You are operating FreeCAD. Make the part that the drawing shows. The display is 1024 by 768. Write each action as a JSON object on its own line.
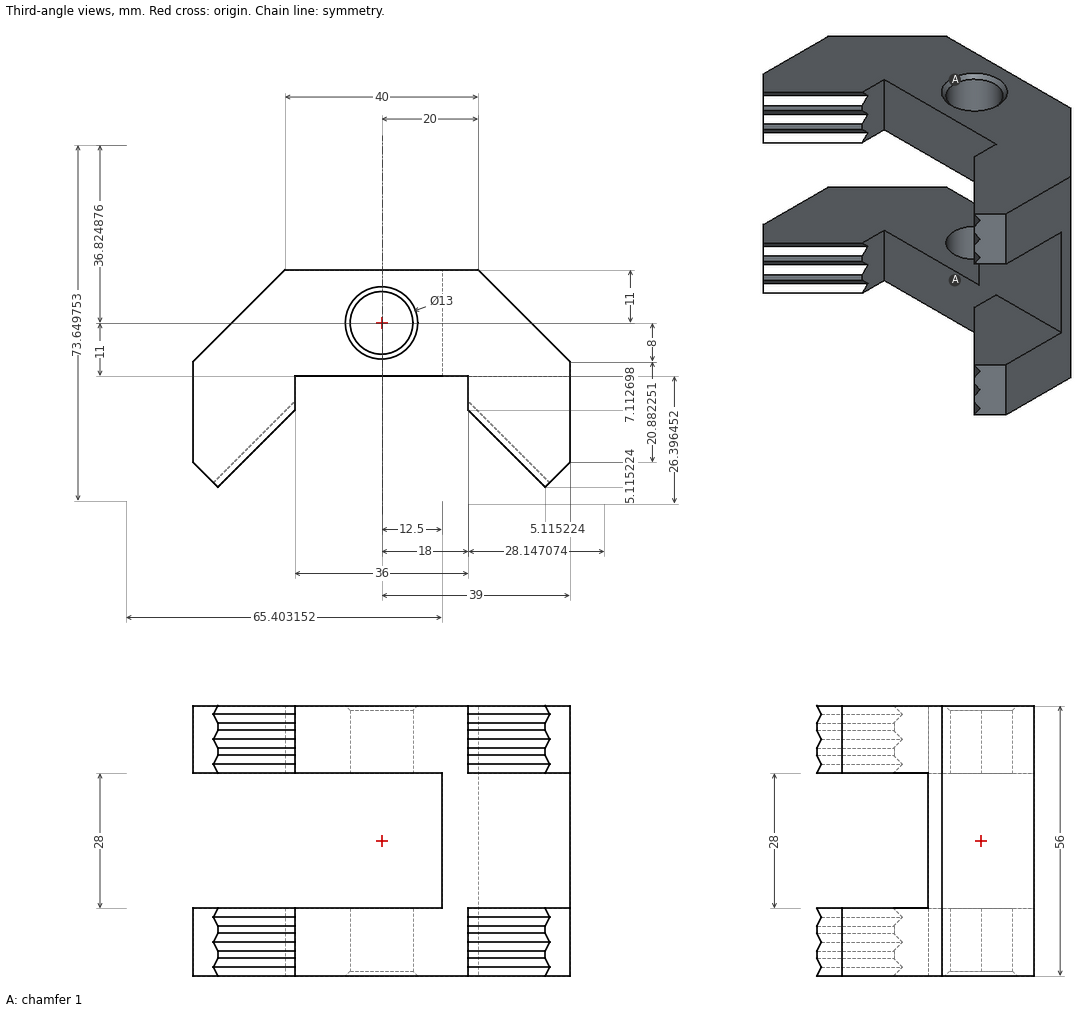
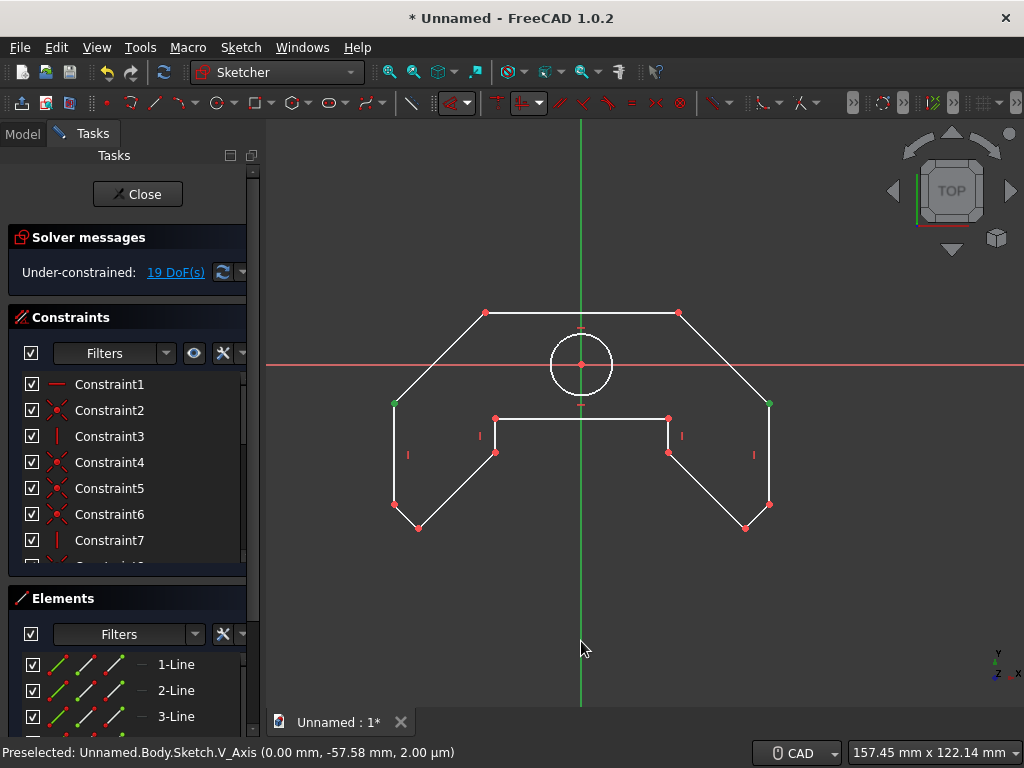
{"action": "left_click", "coordinate": [656, 104]}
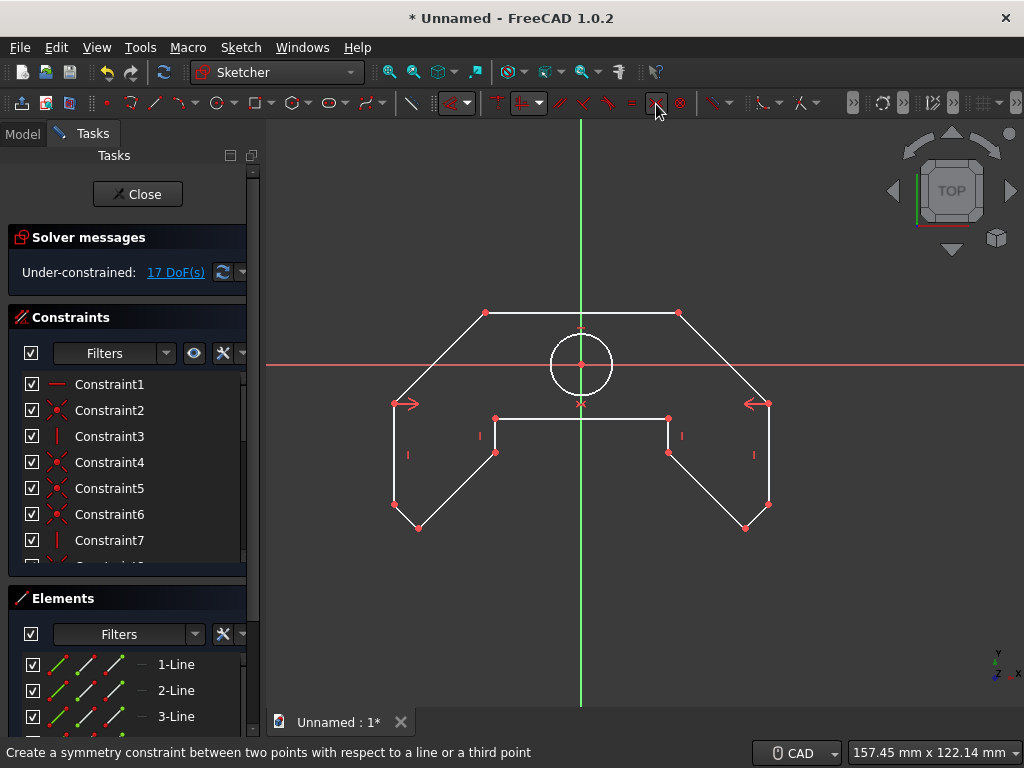
{"action": "left_click", "coordinate": [745, 529]}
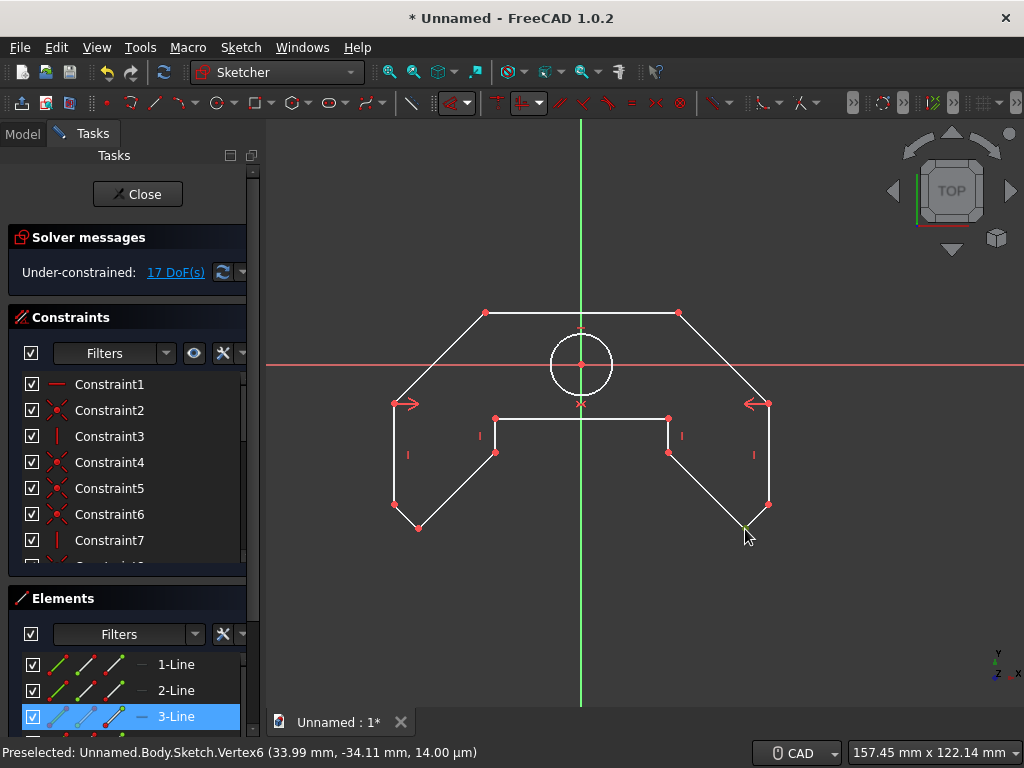
{"action": "left_click", "coordinate": [418, 529]}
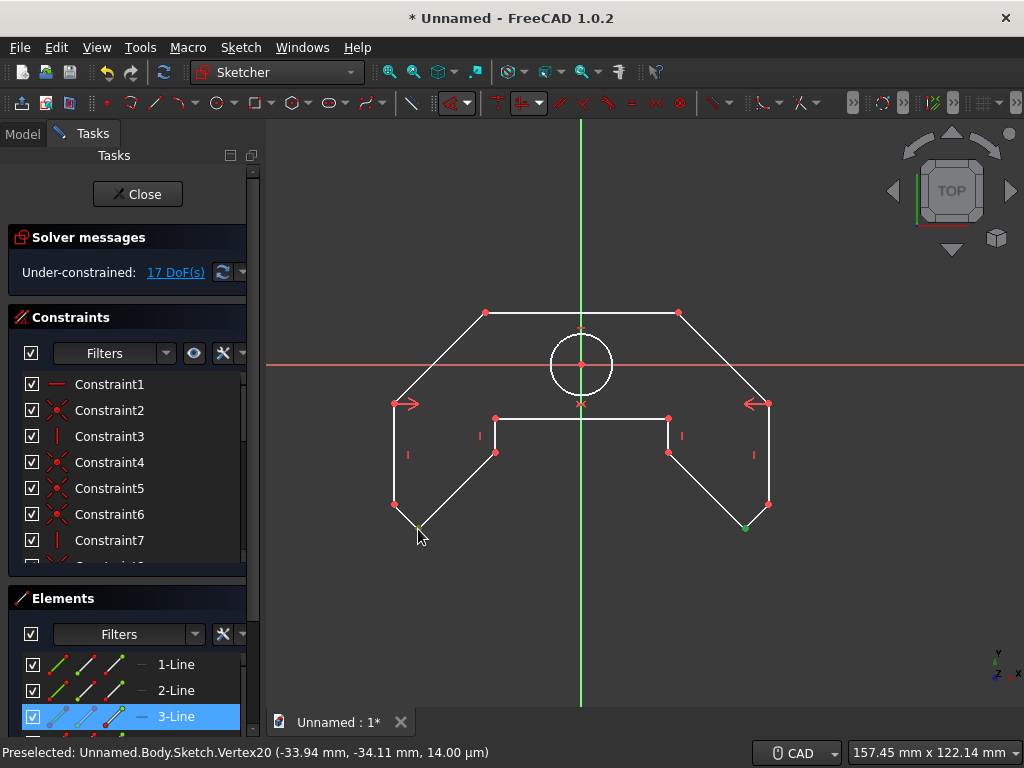
{"action": "left_click", "coordinate": [581, 641]}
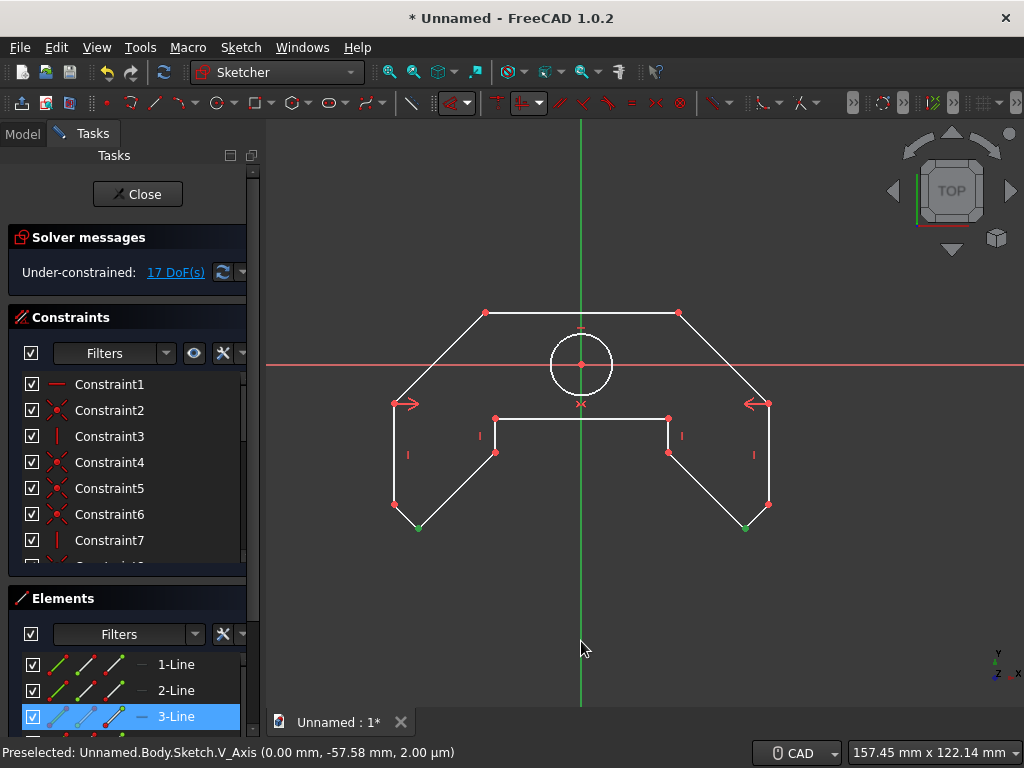
{"action": "key", "text": "s"}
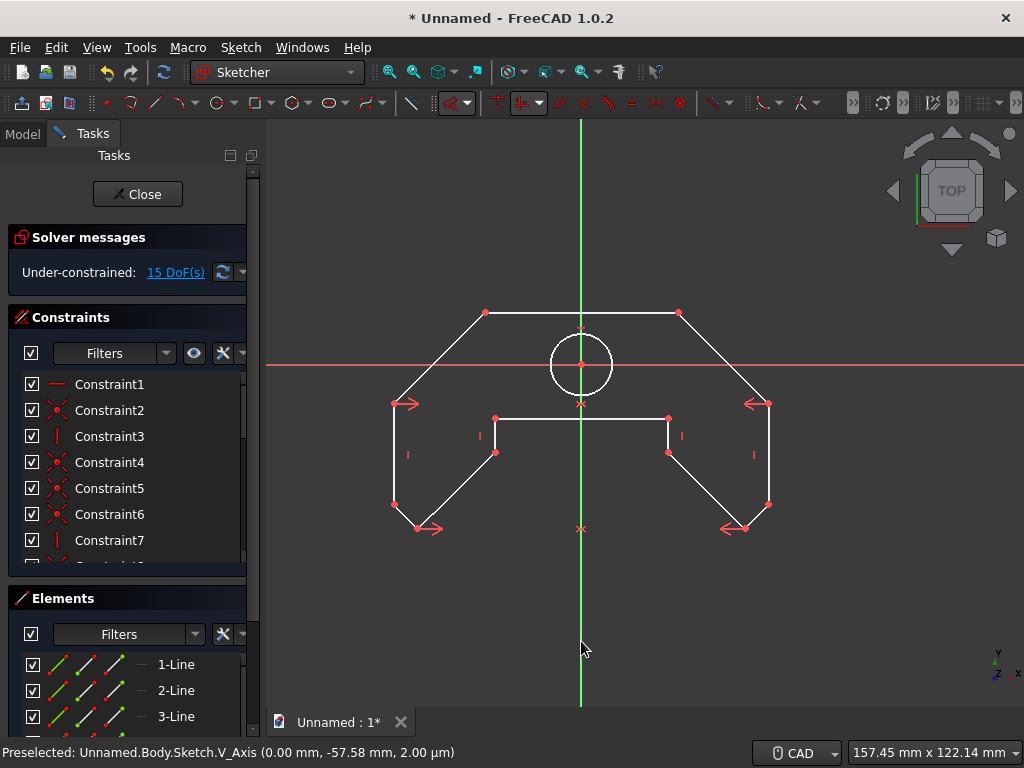
{"action": "left_click", "coordinate": [668, 453]}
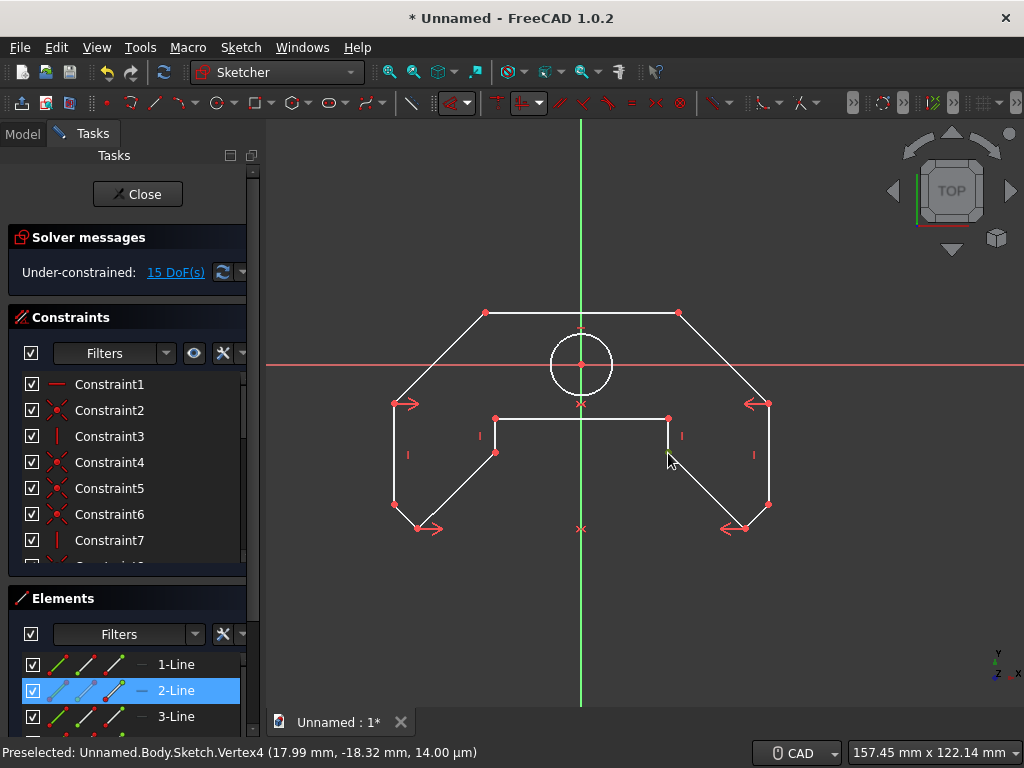
{"action": "left_click", "coordinate": [495, 453]}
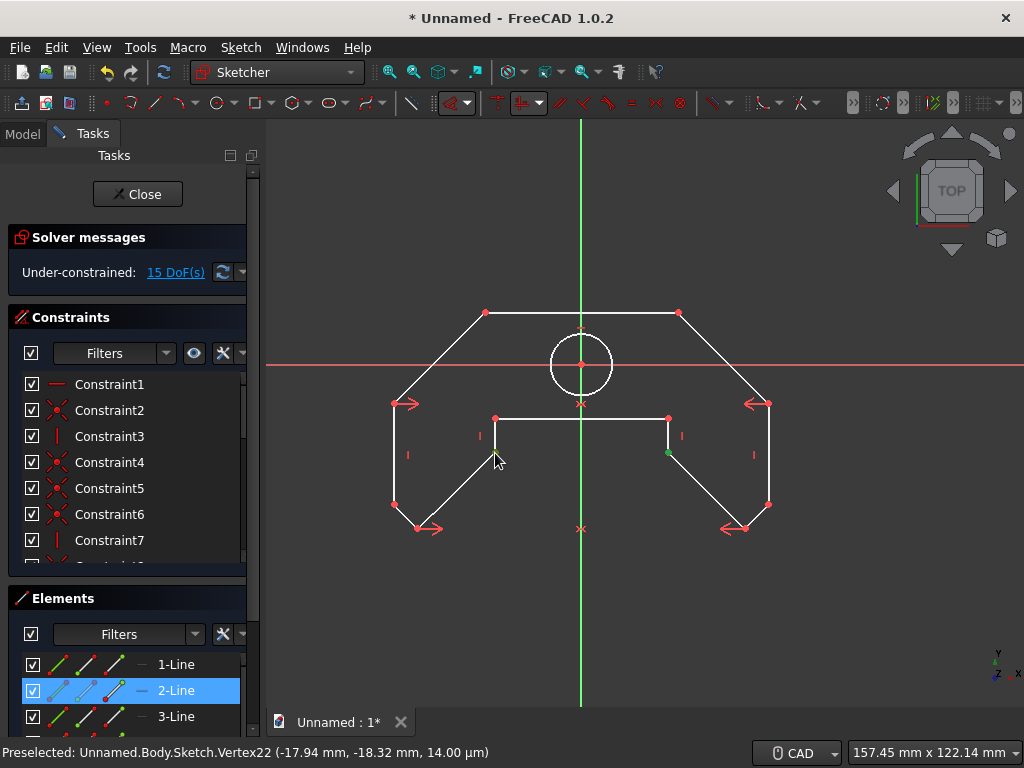
{"action": "left_click", "coordinate": [581, 641]}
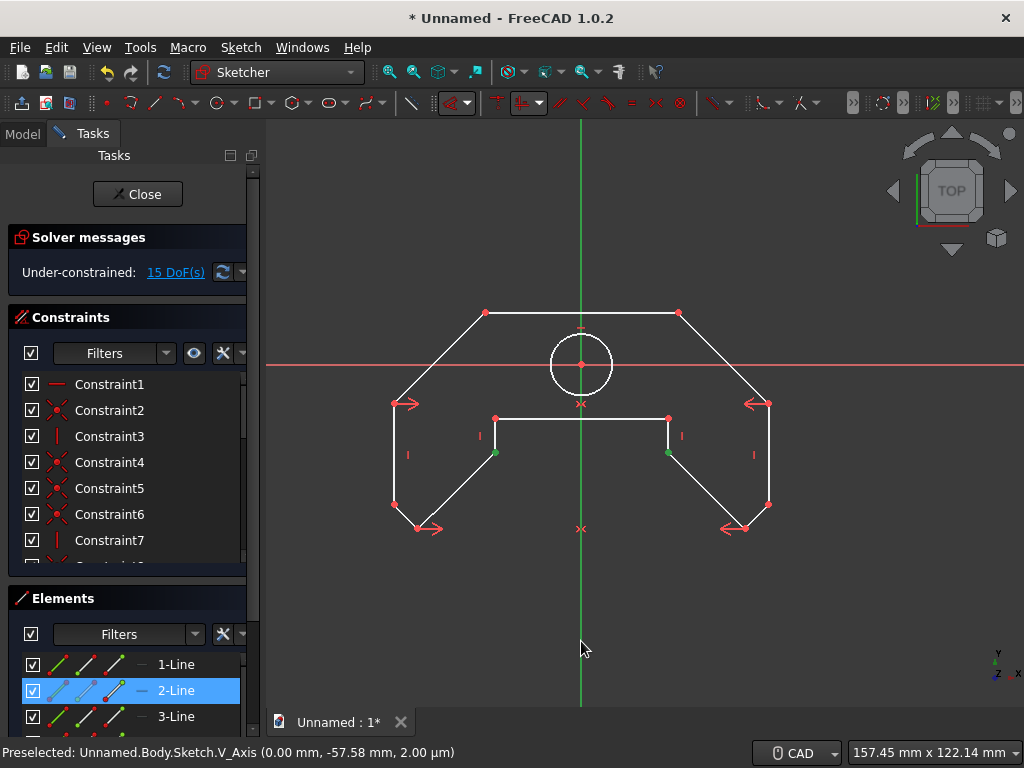
{"action": "key", "text": "s"}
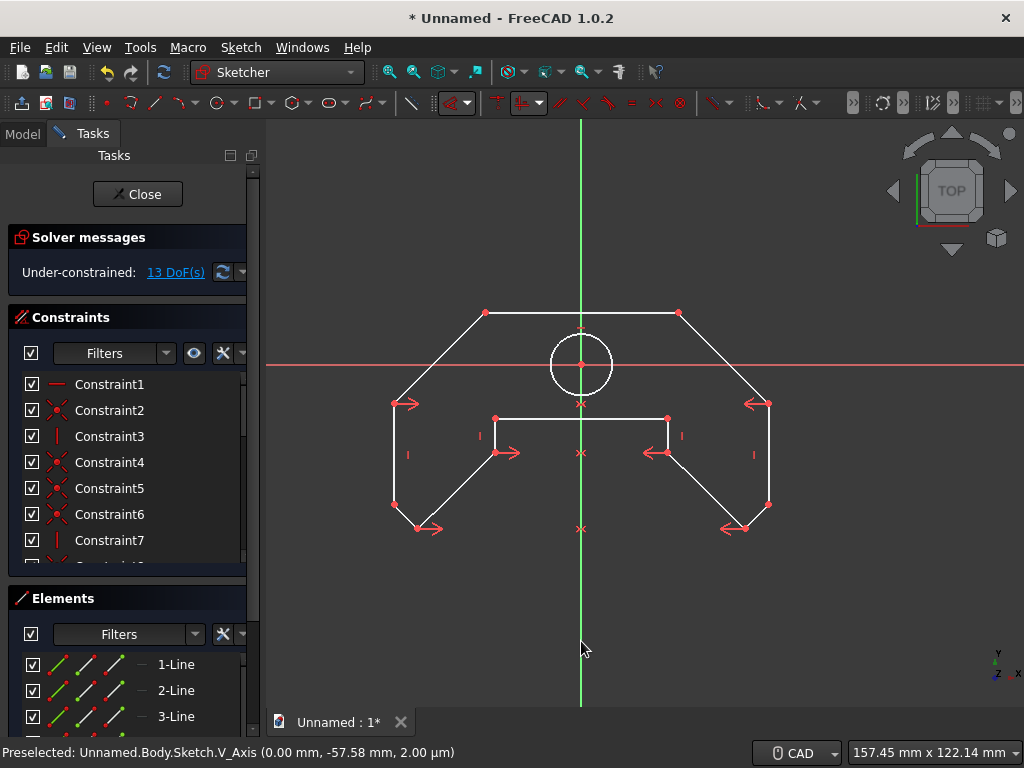
{"action": "left_click", "coordinate": [603, 343]}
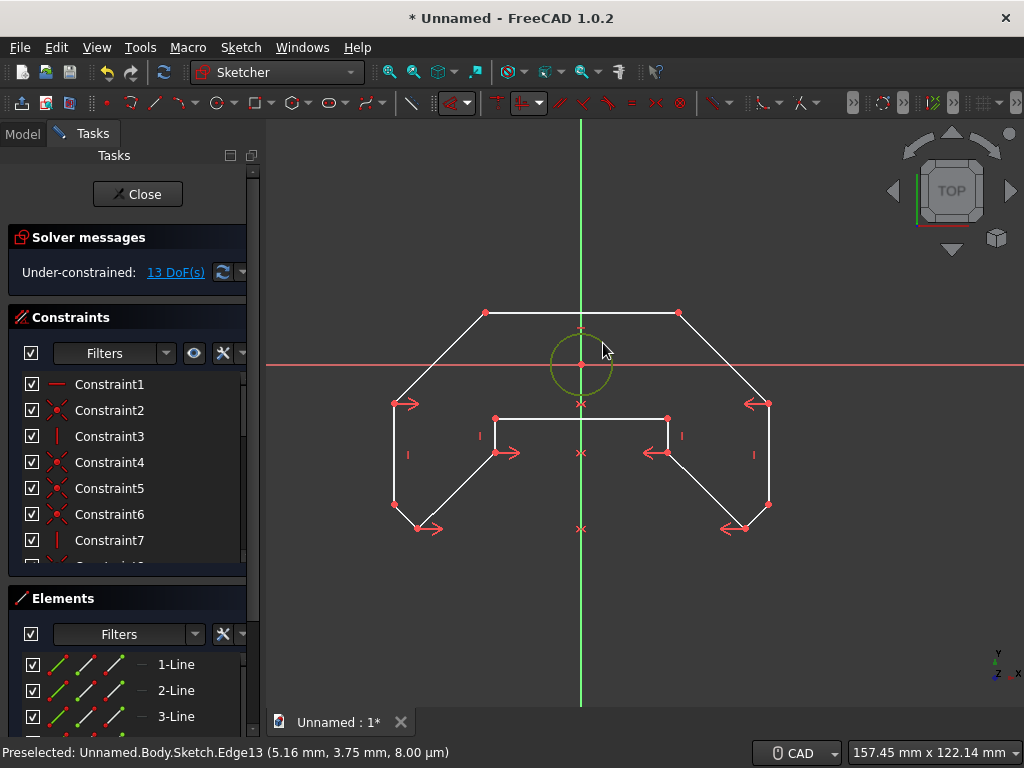
{"action": "left_click", "coordinate": [470, 104]}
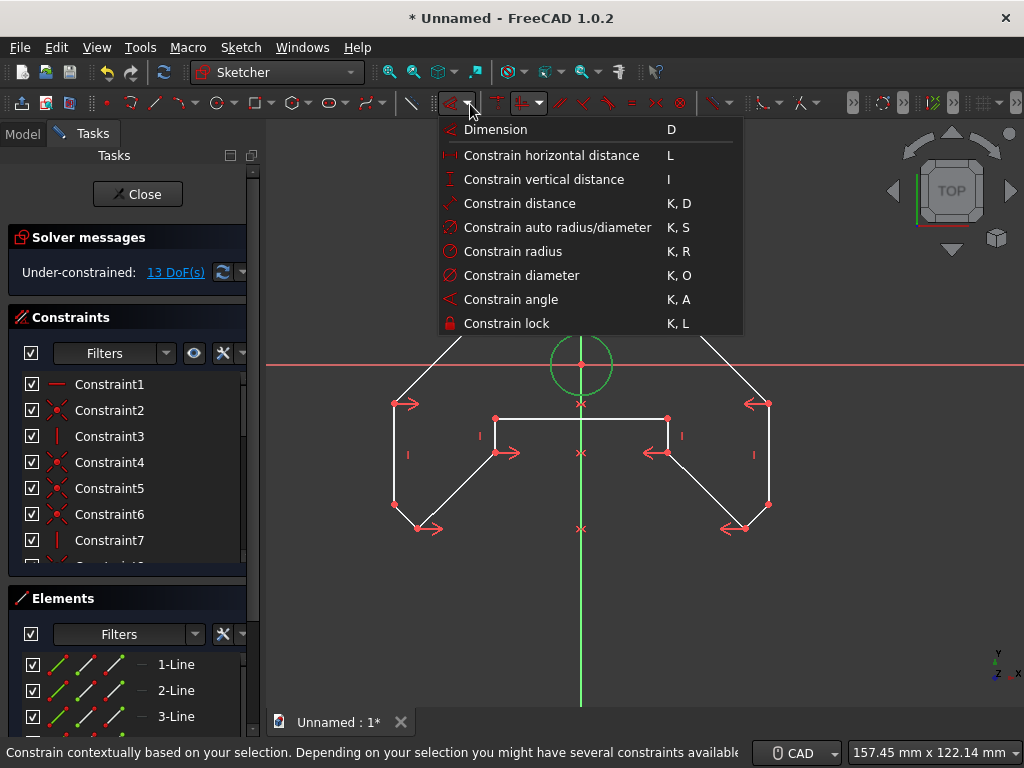
{"action": "left_click", "coordinate": [591, 275]}